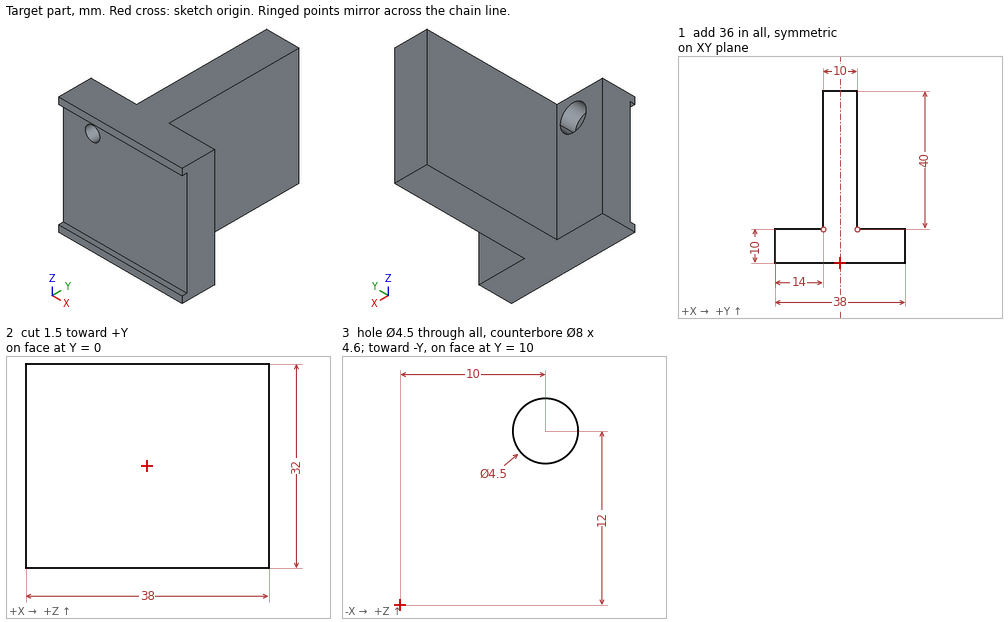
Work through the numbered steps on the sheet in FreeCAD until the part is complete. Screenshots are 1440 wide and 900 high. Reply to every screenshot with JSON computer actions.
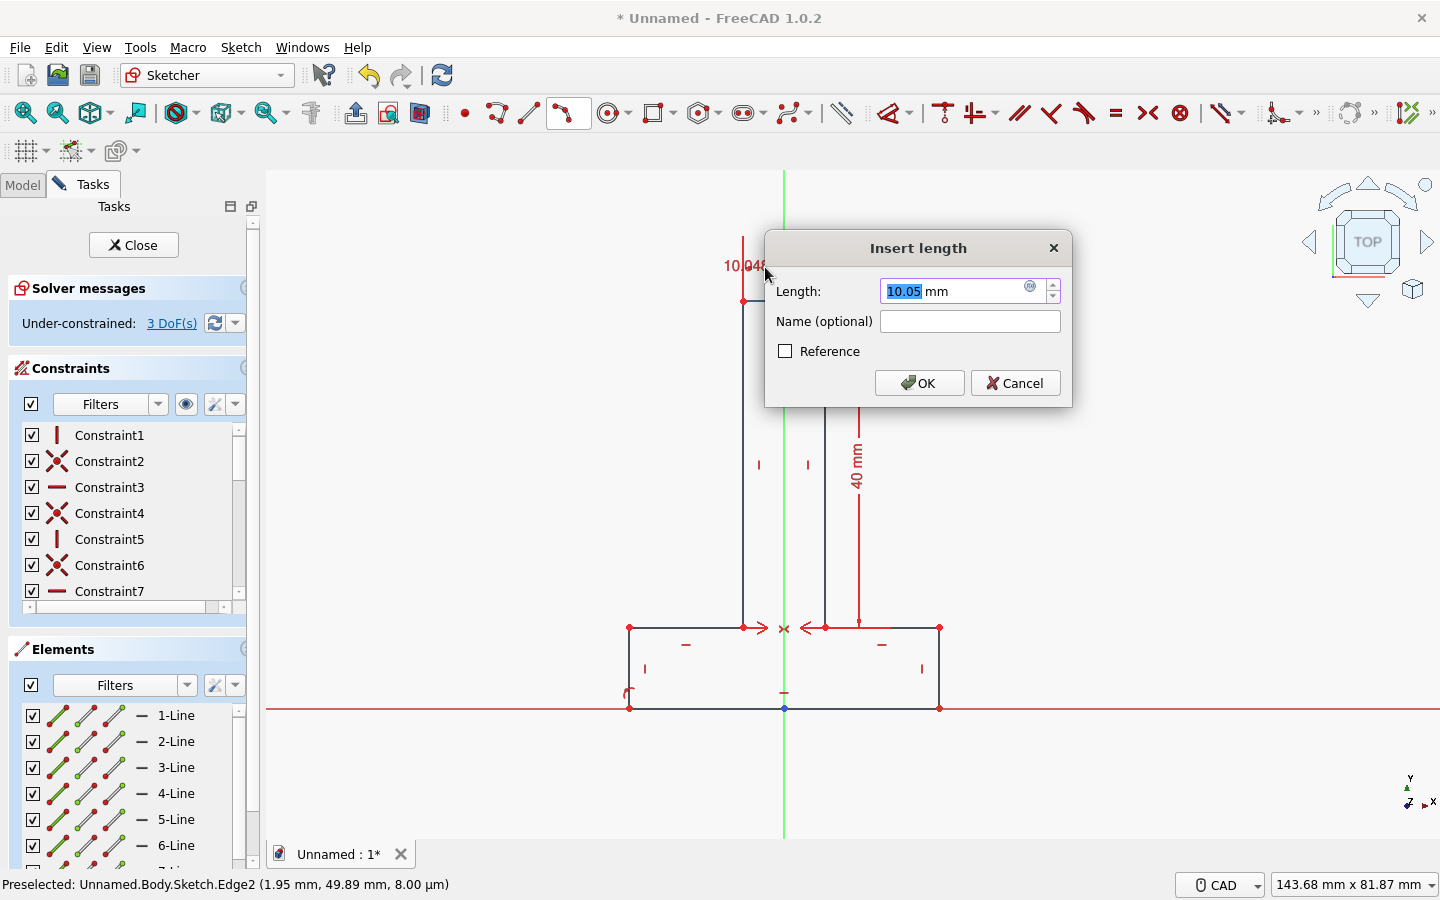
{"action": "type", "text": "10"}
{"action": "key", "text": "Return"}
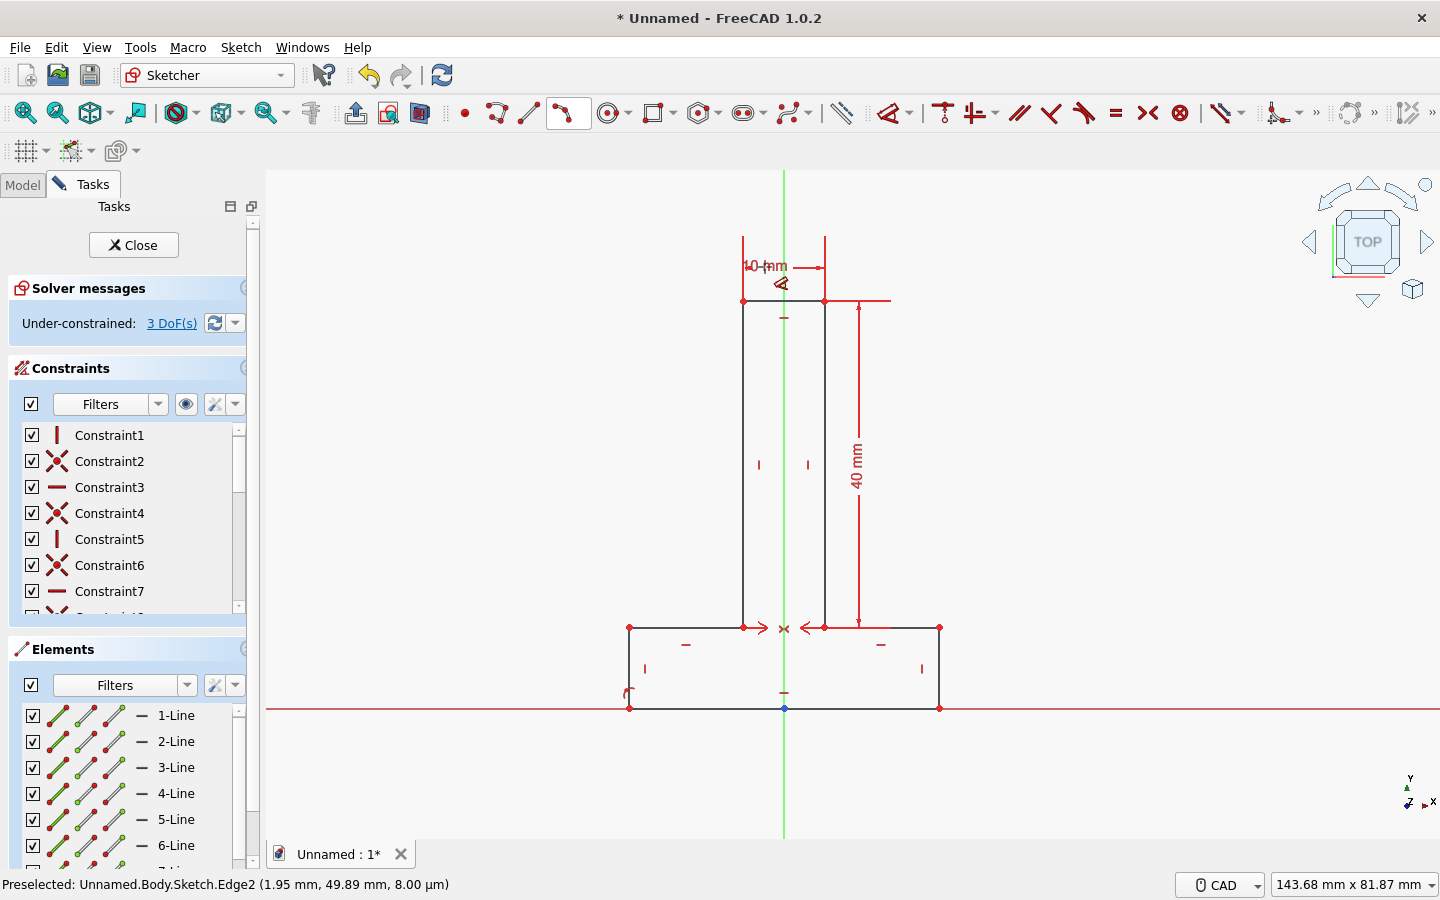
{"action": "left_click", "coordinate": [709, 628]}
{"action": "left_click", "coordinate": [686, 662]}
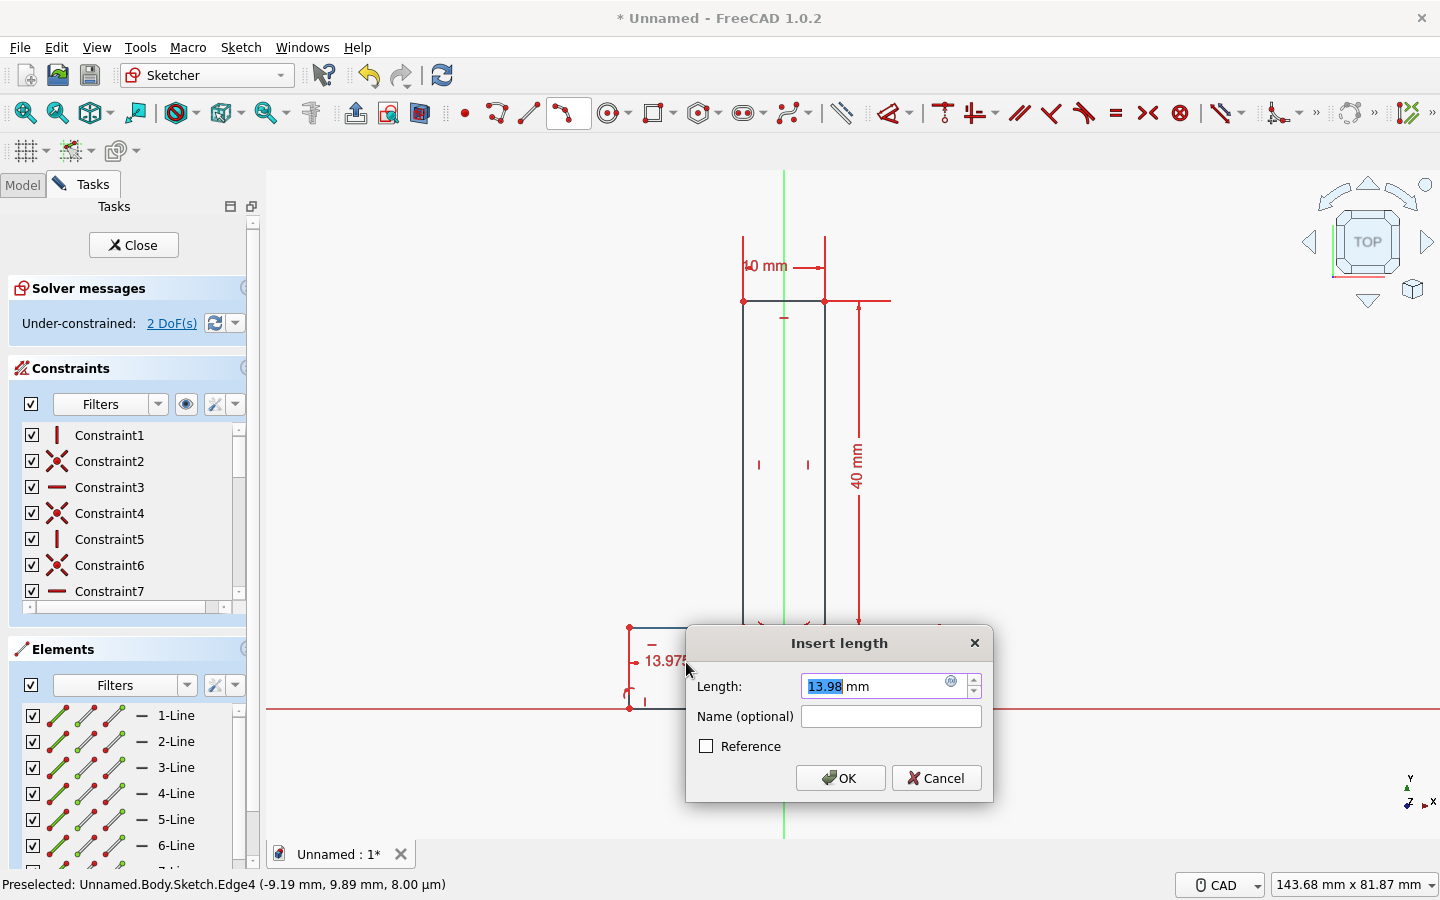
{"action": "type", "text": "14"}
{"action": "key", "text": "Return"}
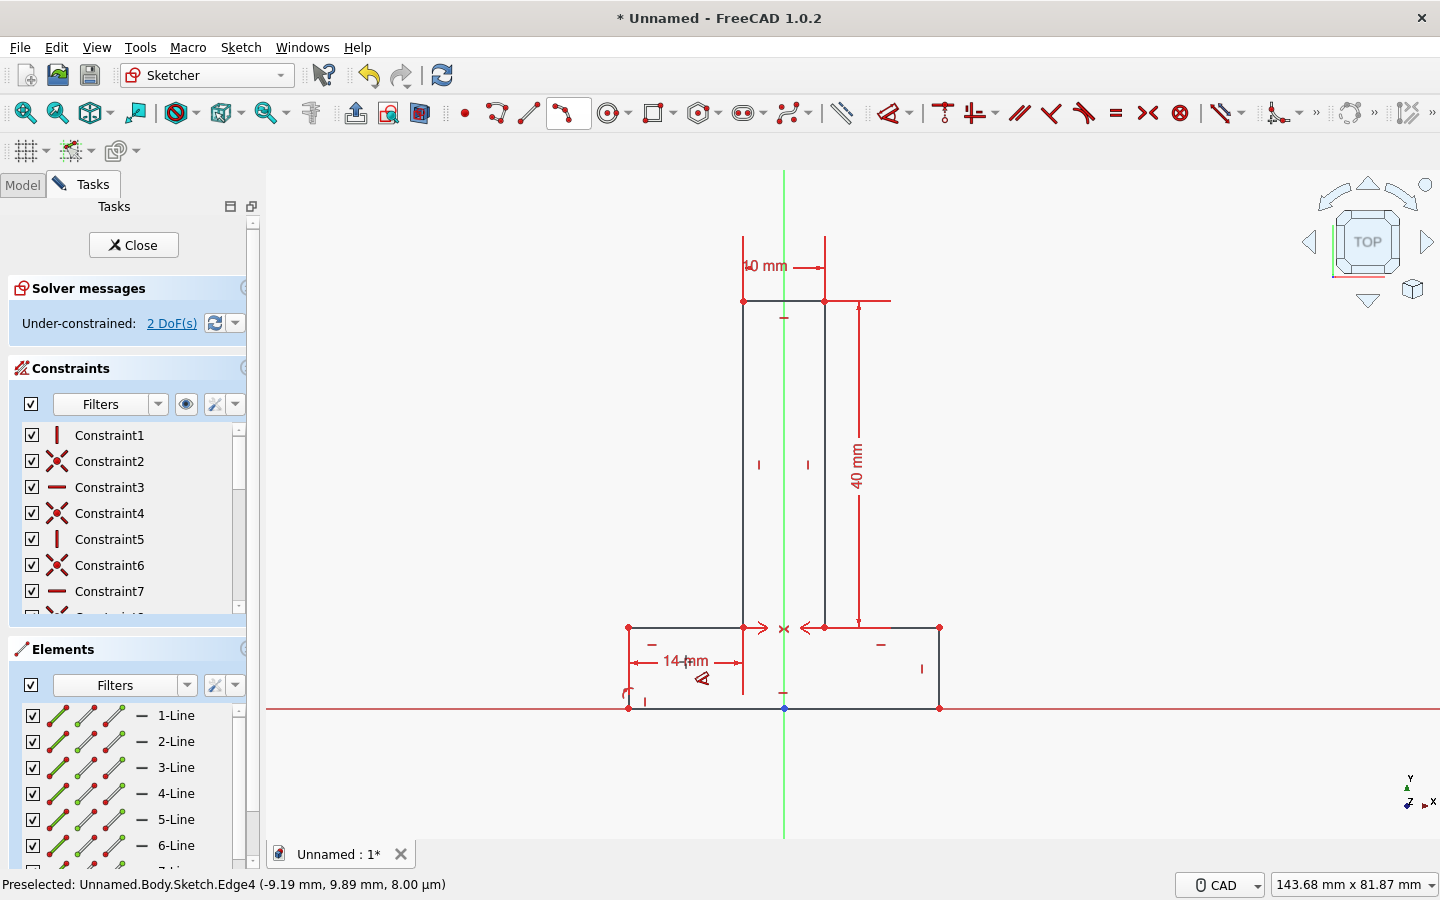
{"action": "left_click", "coordinate": [629, 652]}
{"action": "left_click", "coordinate": [595, 668]}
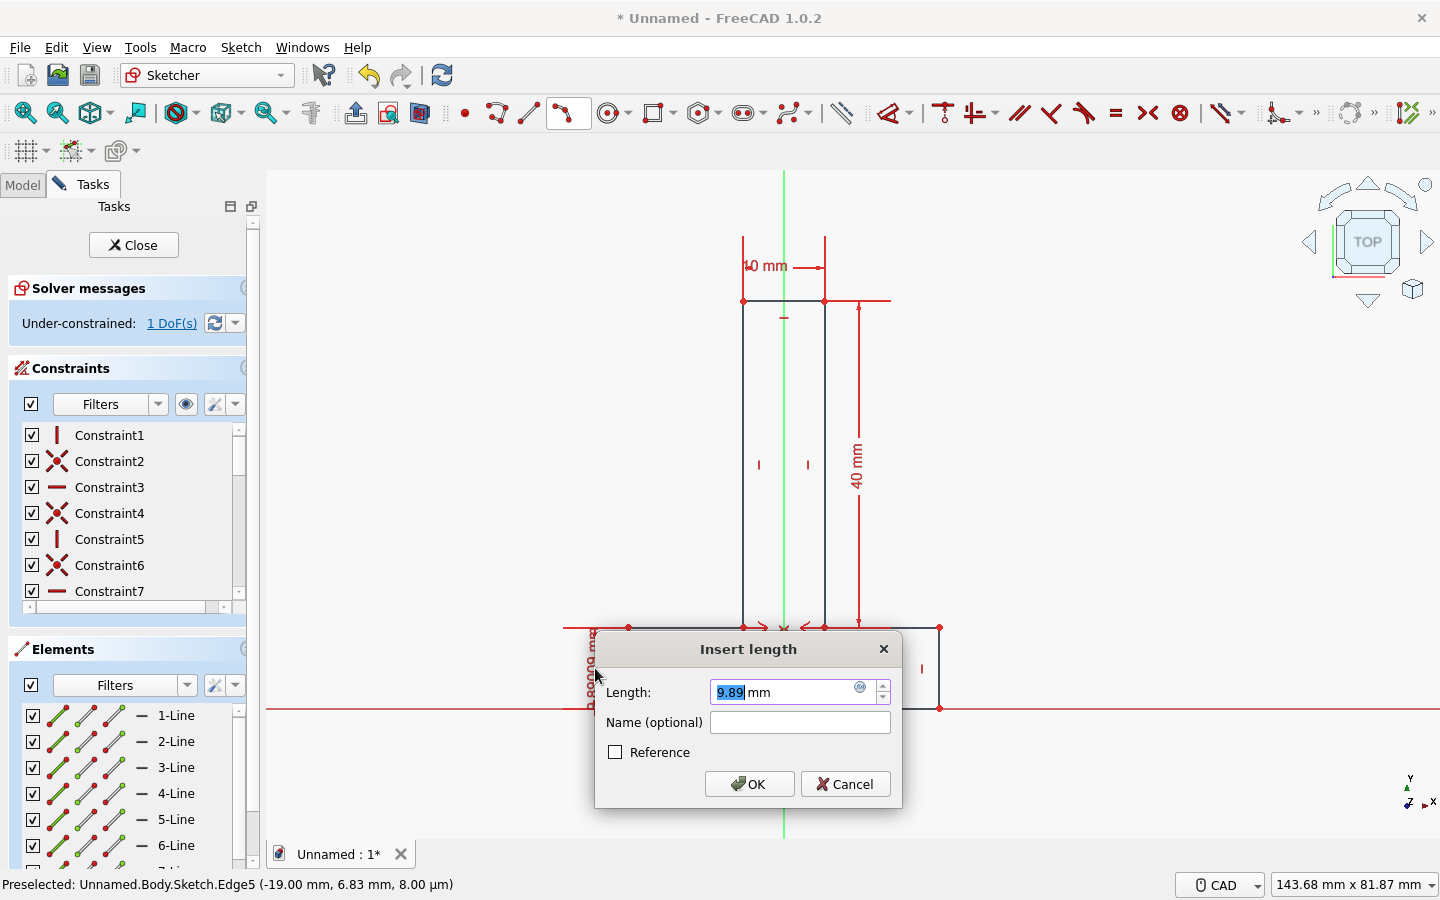
{"action": "type", "text": "10"}
{"action": "key", "text": "Return"}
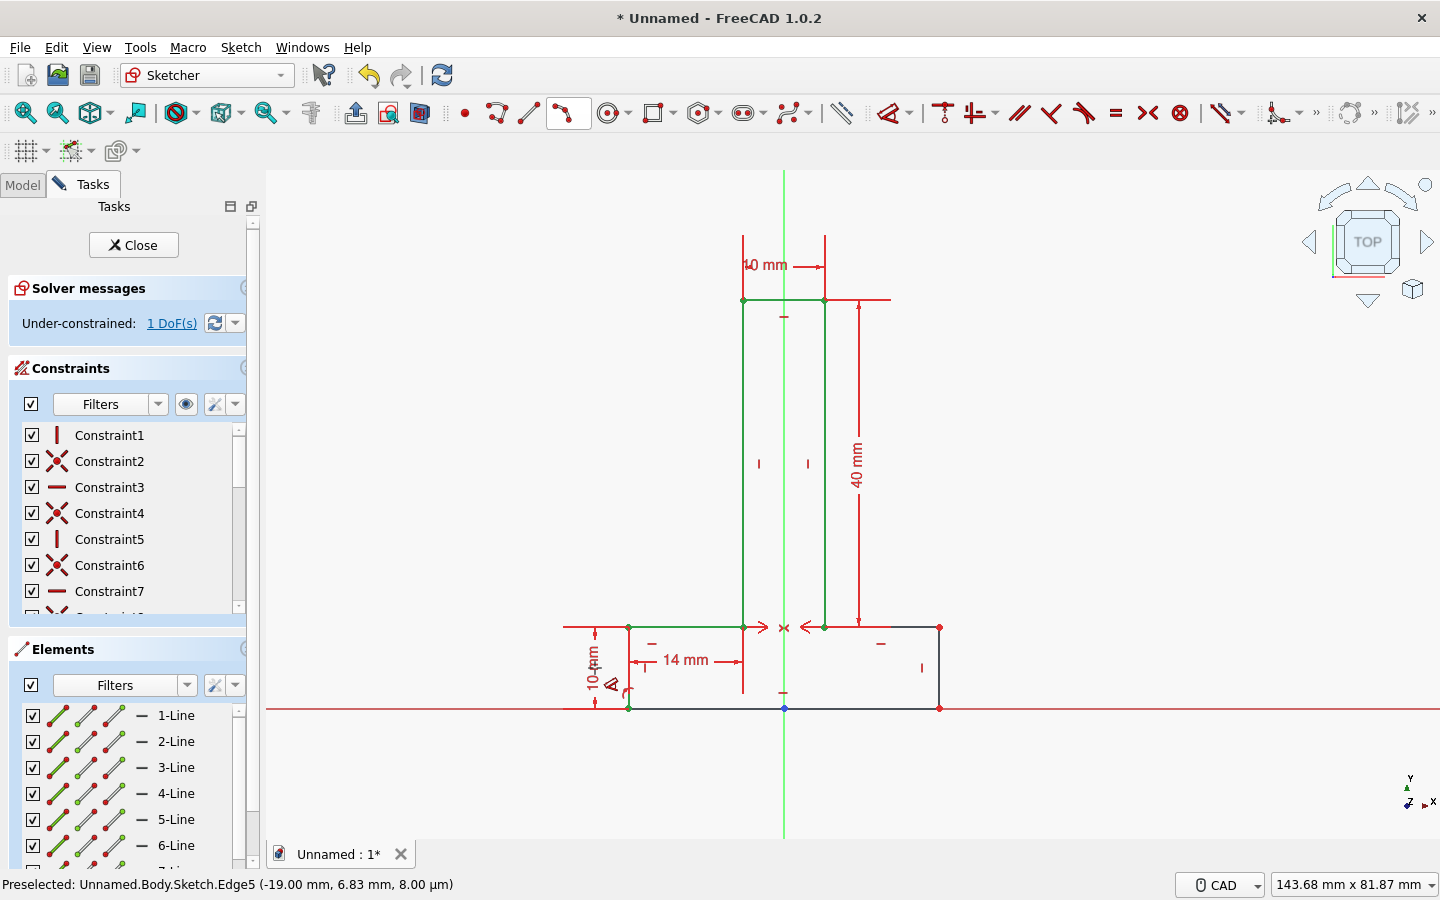
{"action": "left_click", "coordinate": [722, 709]}
{"action": "left_click", "coordinate": [713, 743]}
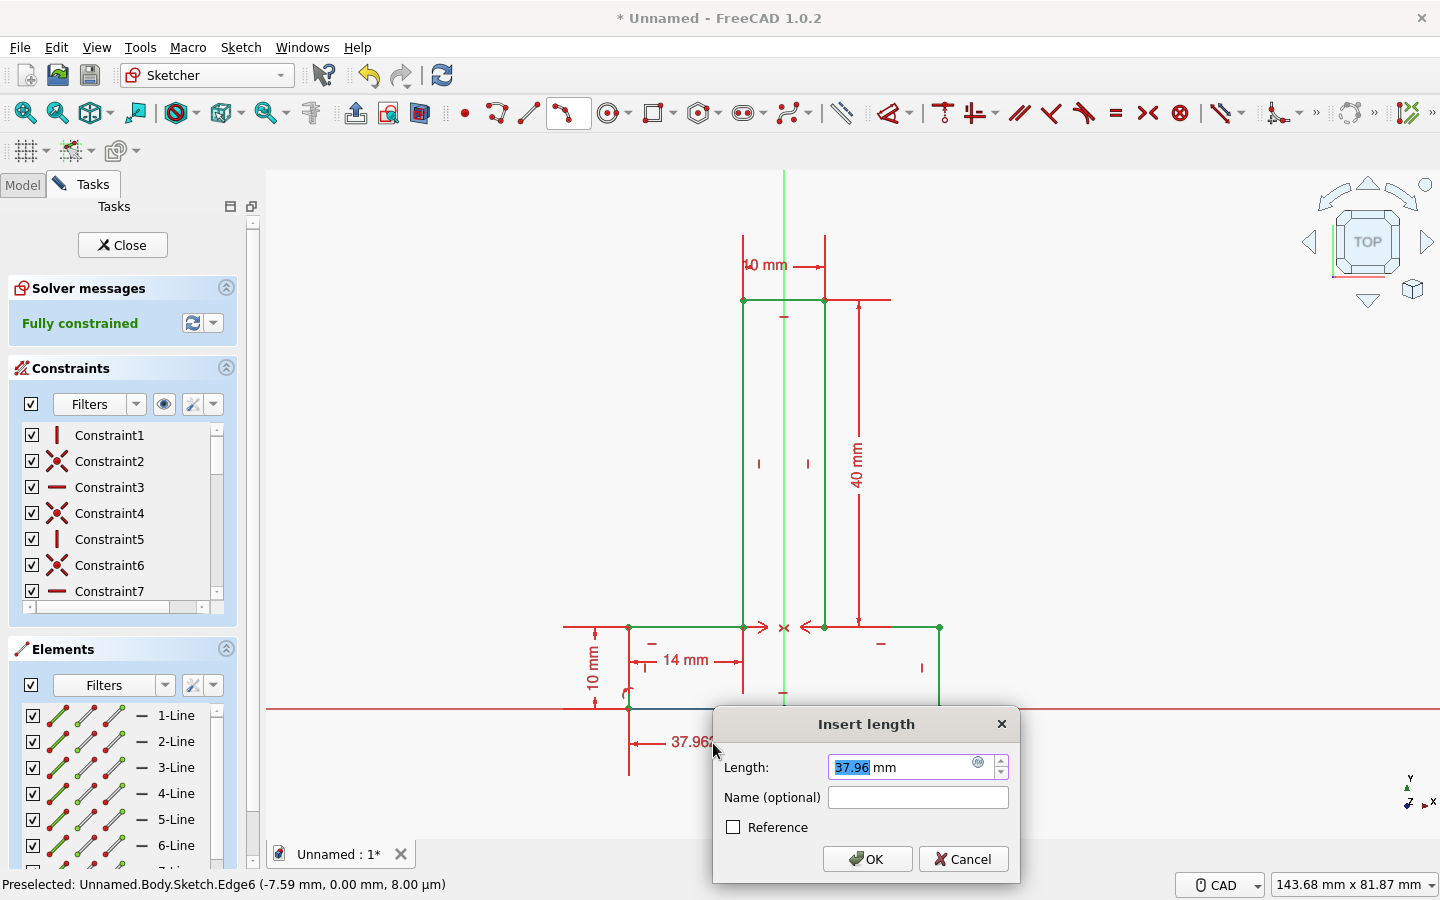
{"action": "type", "text": "38"}
{"action": "key", "text": "Return"}
{"action": "key", "text": "Escape"}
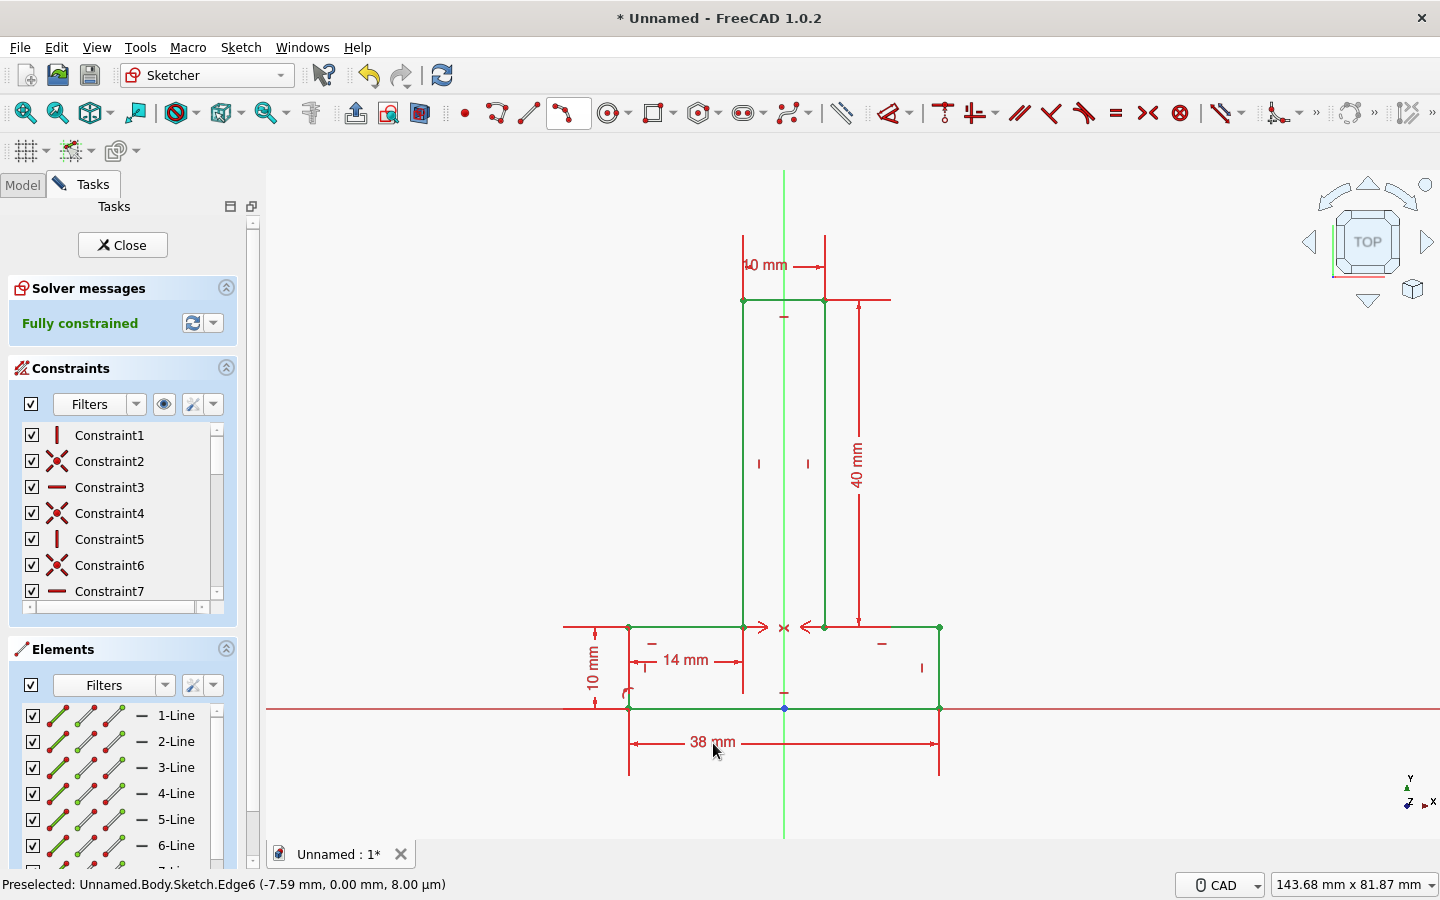
{"action": "left_click", "coordinate": [123, 245]}